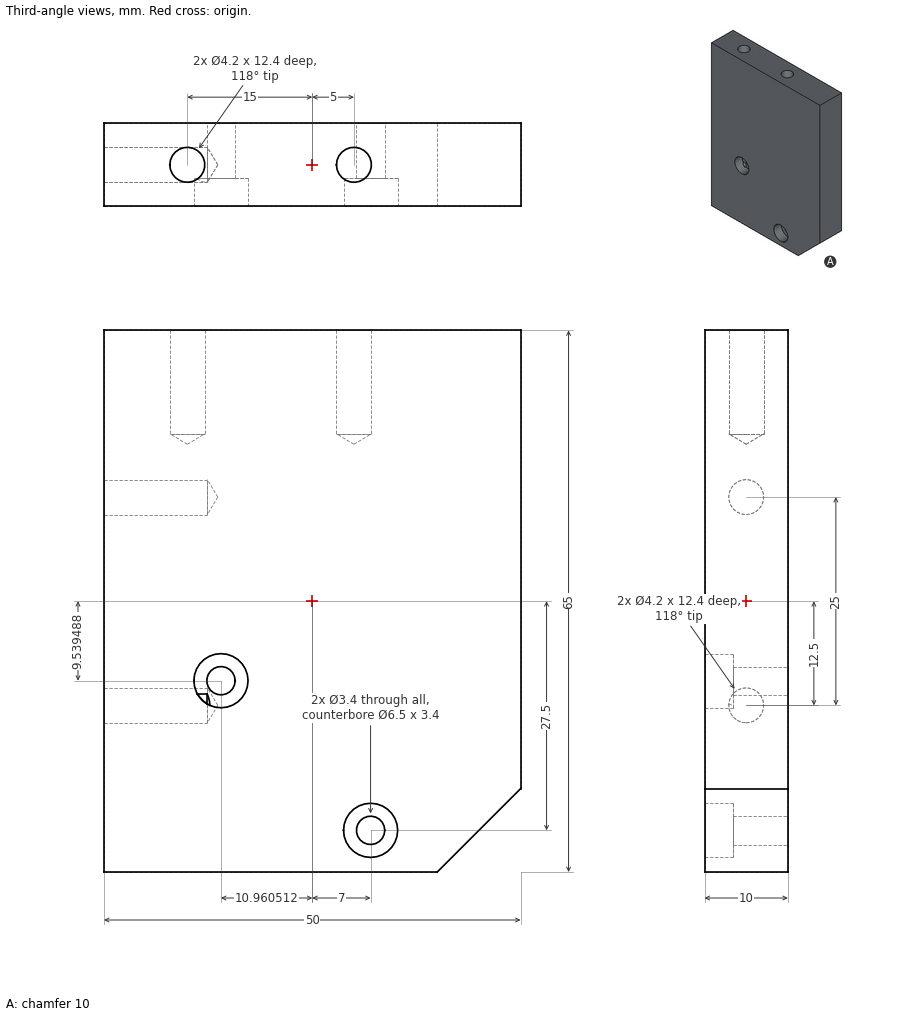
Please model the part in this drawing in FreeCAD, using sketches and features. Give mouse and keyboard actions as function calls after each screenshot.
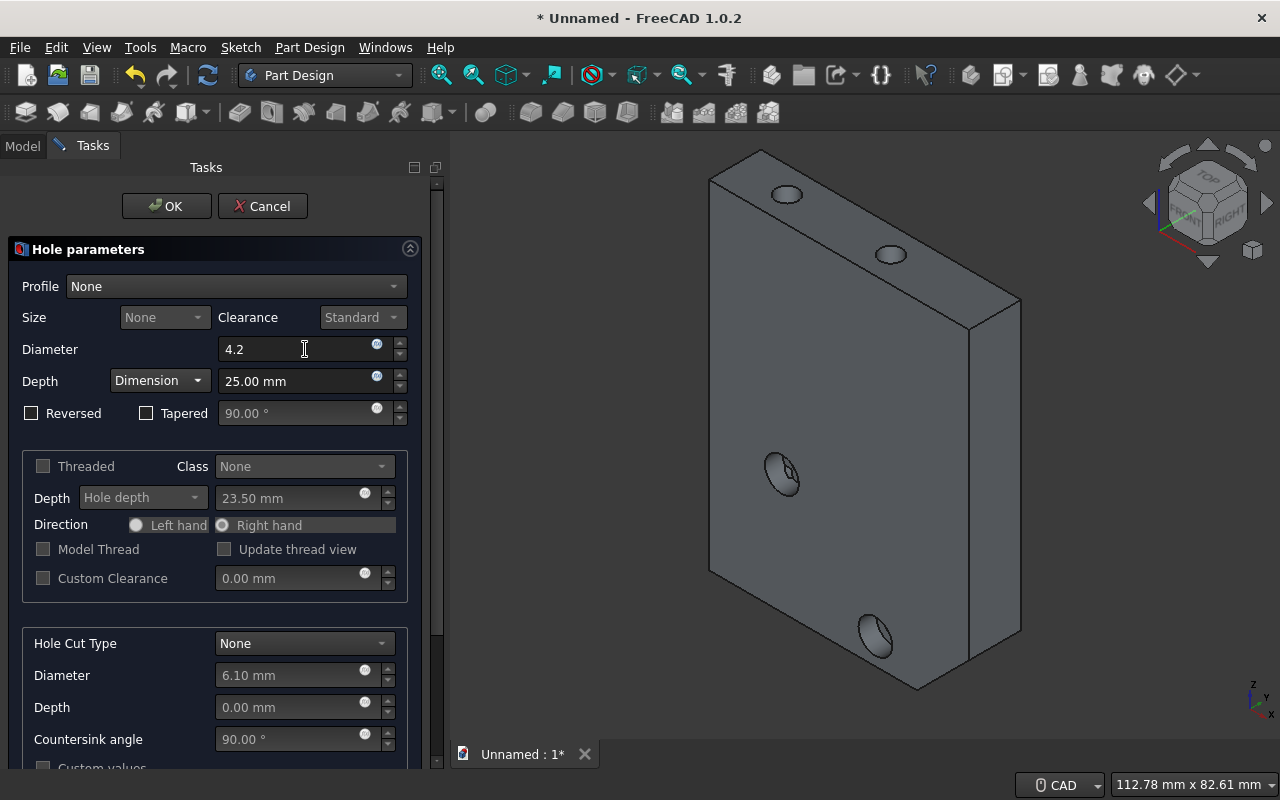
triple_click(305, 381)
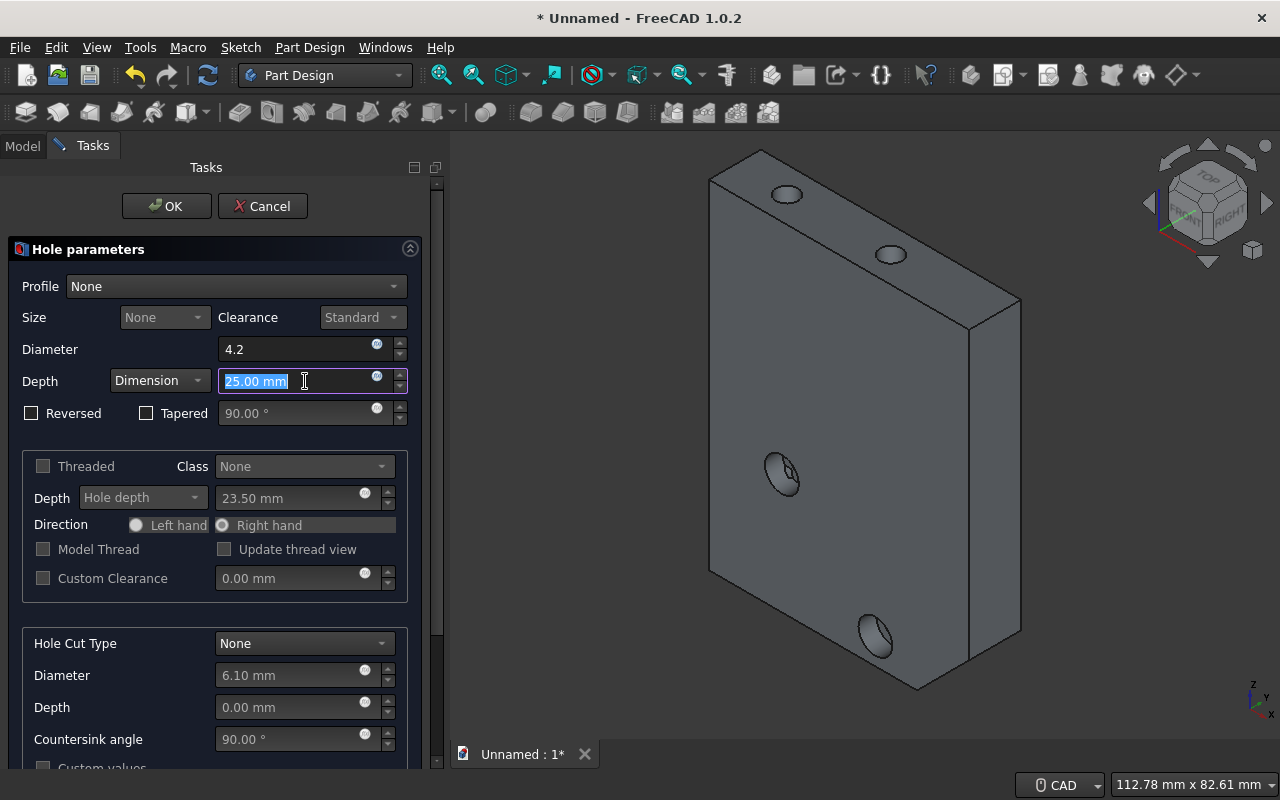
text(12.4)
key(Tab)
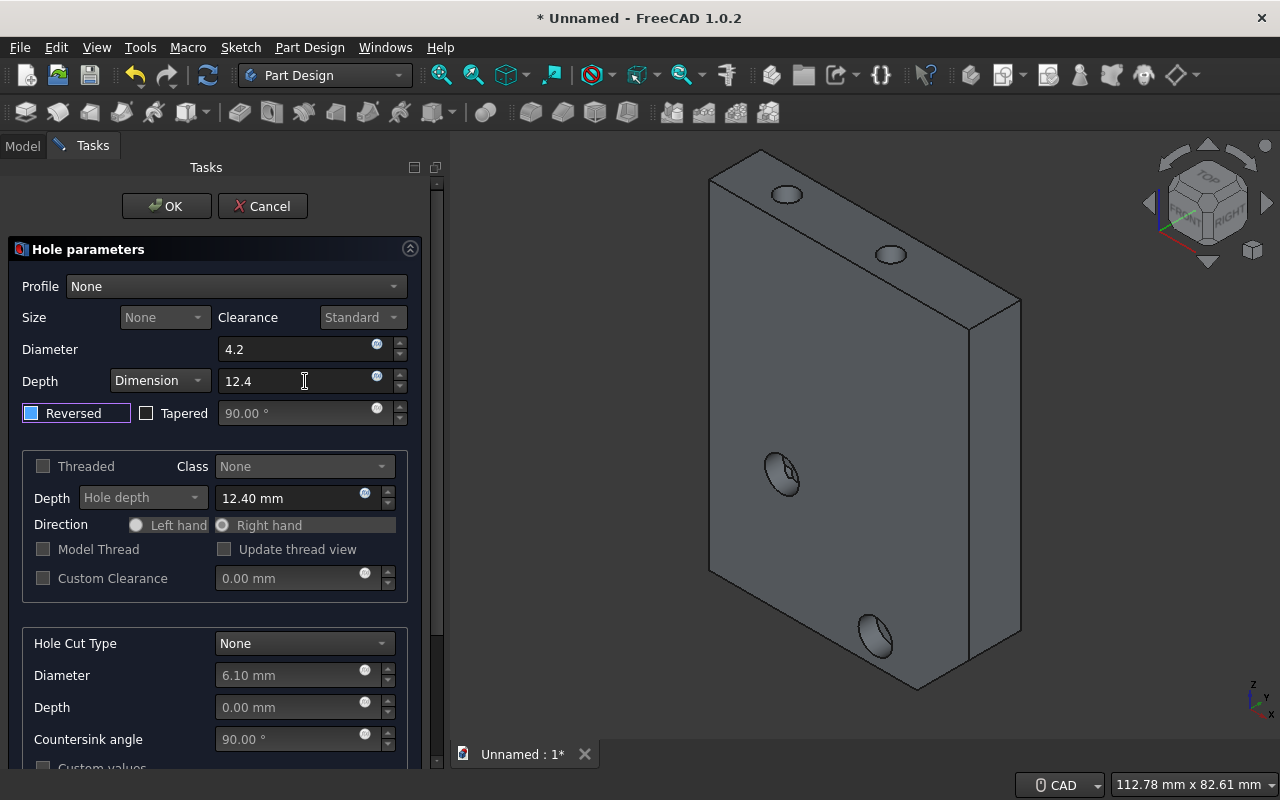
click(167, 206)